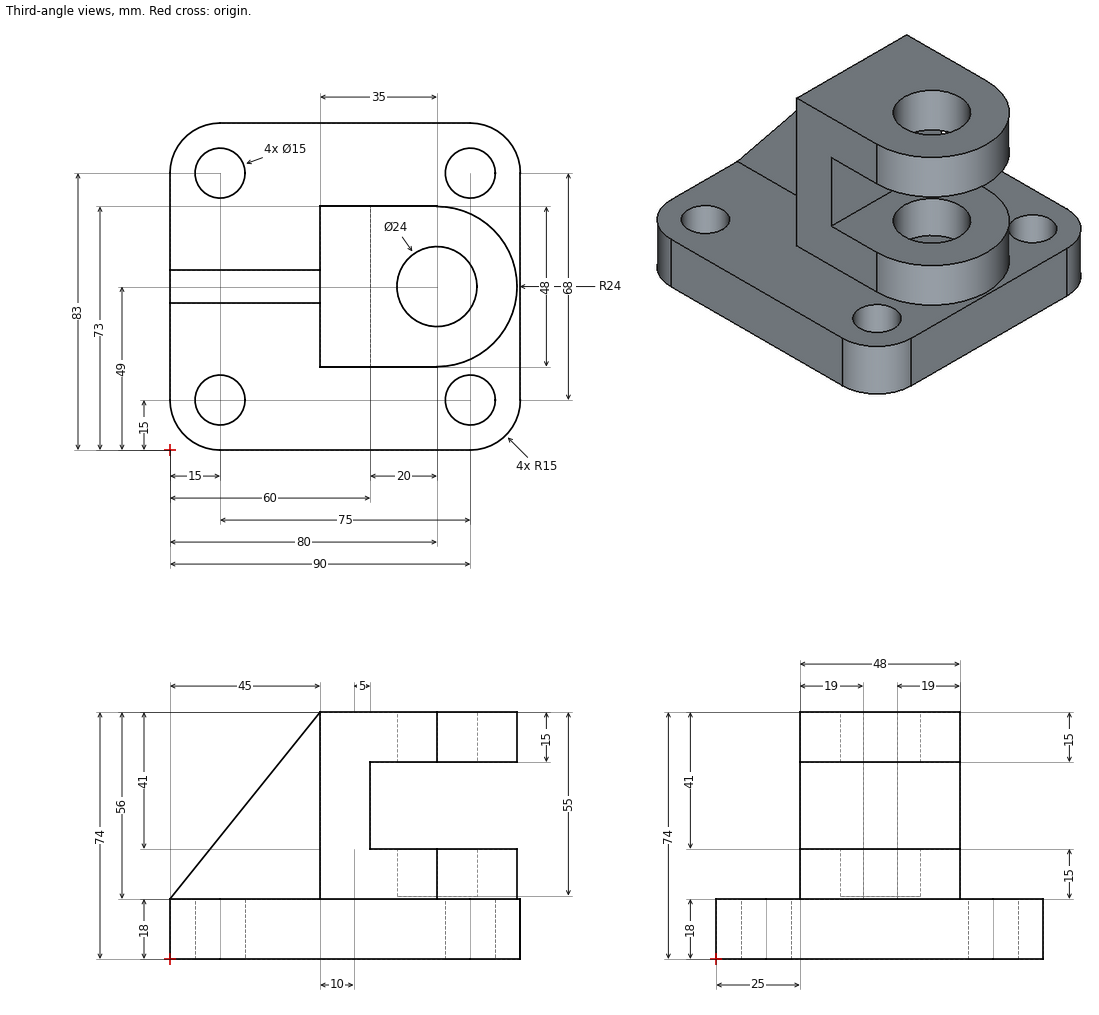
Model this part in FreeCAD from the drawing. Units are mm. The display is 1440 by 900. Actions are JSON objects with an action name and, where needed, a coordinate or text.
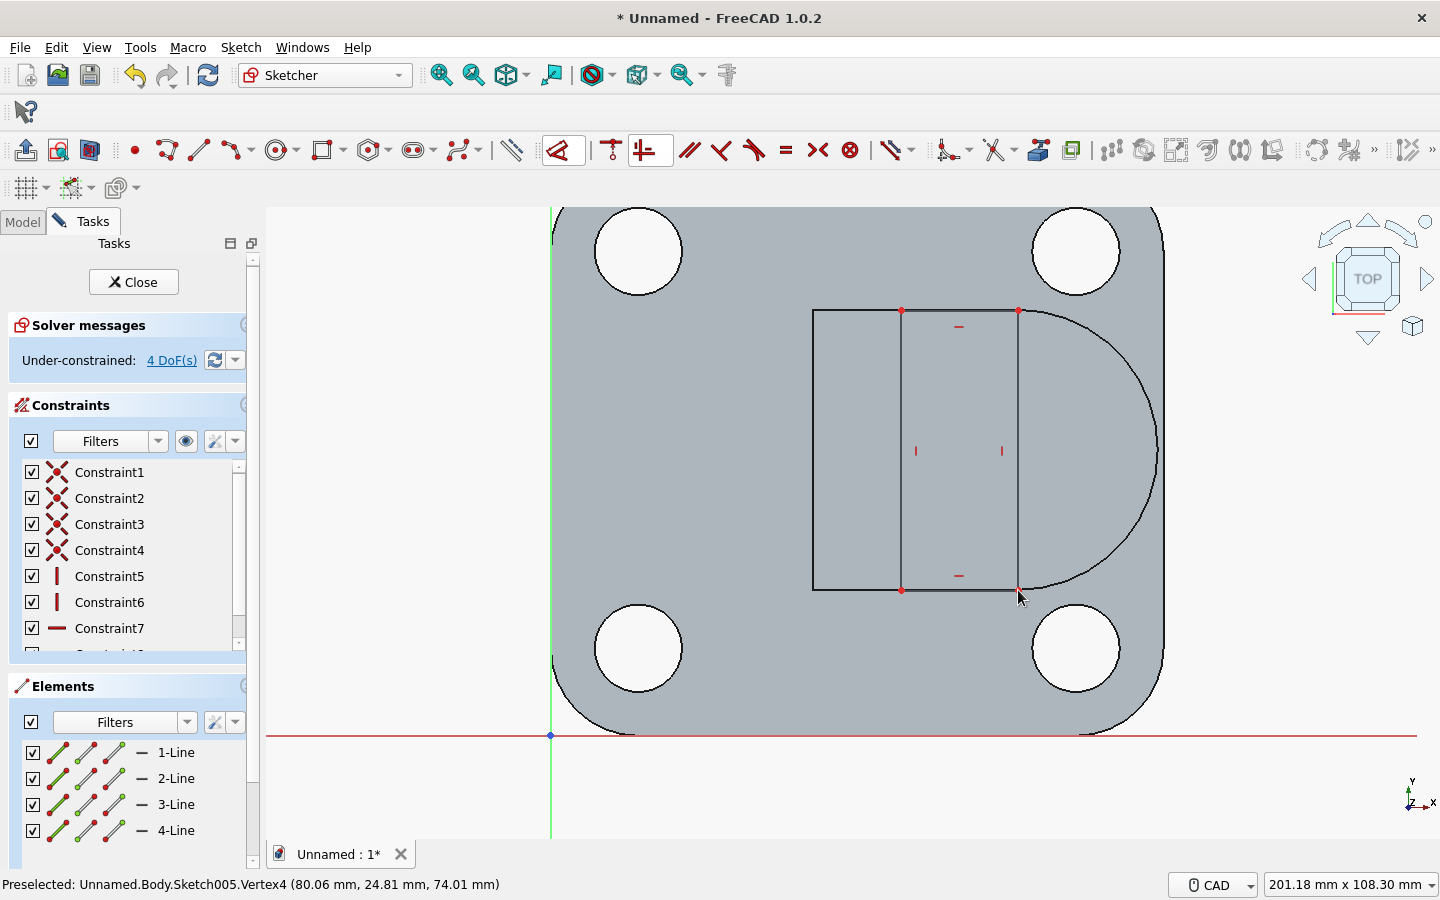
{"action": "left_click", "coordinate": [901, 395]}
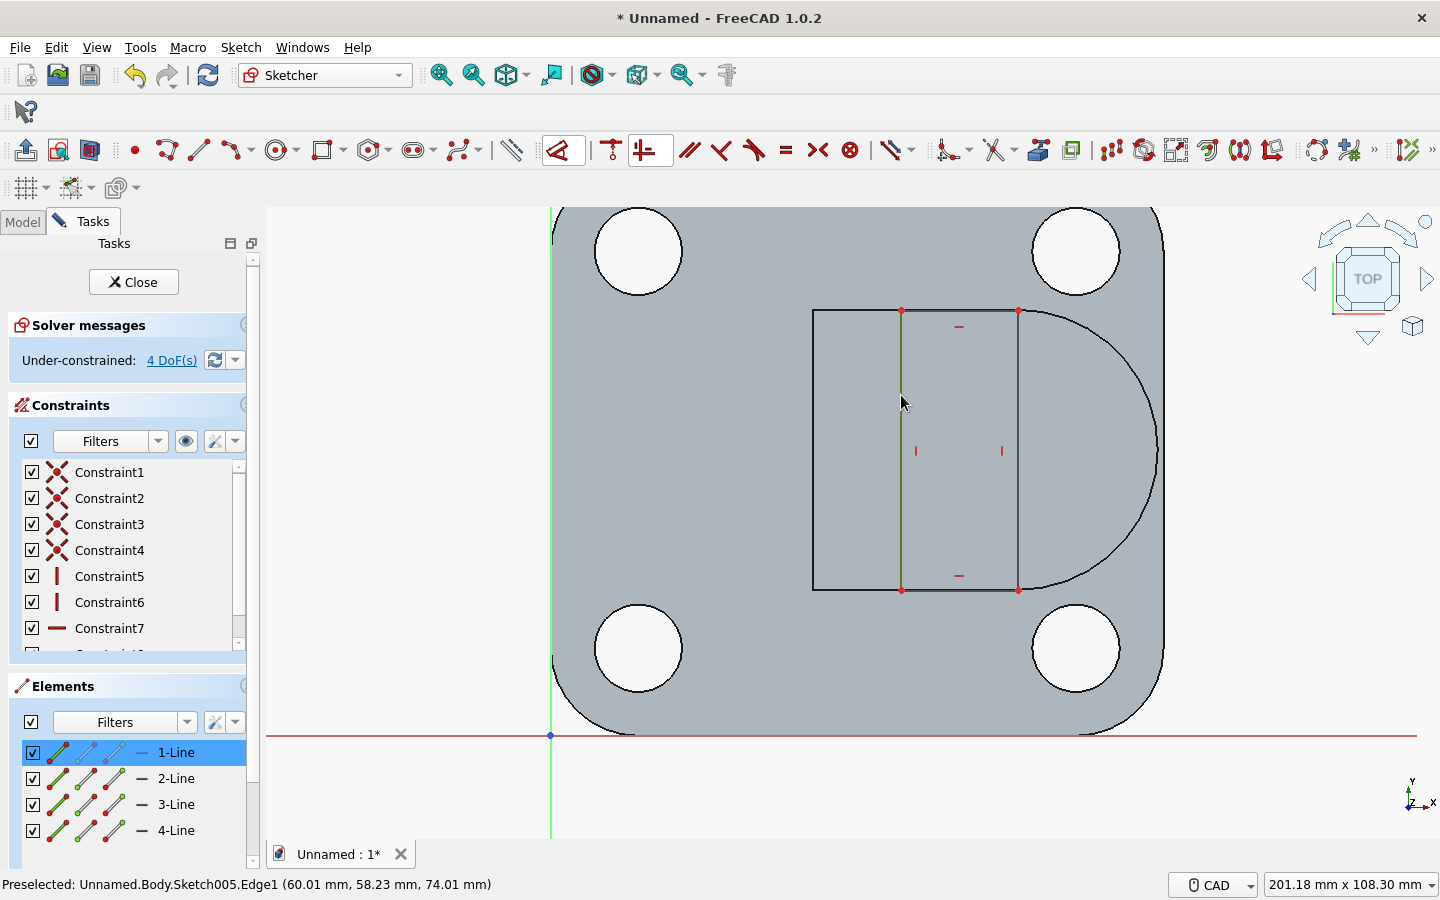
{"action": "left_click", "coordinate": [580, 150]}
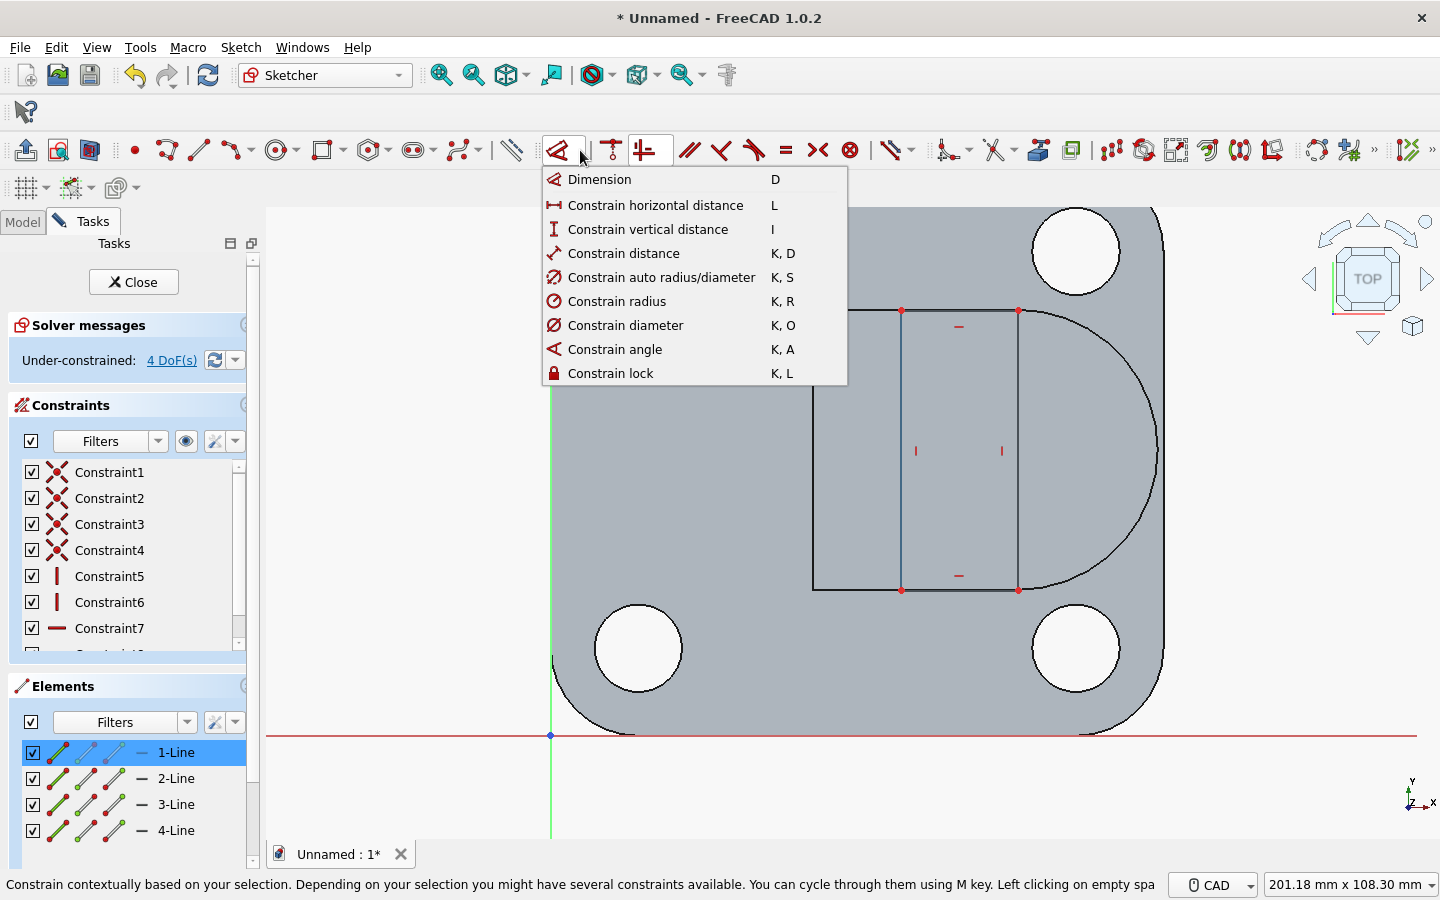
{"action": "left_click", "coordinate": [695, 229]}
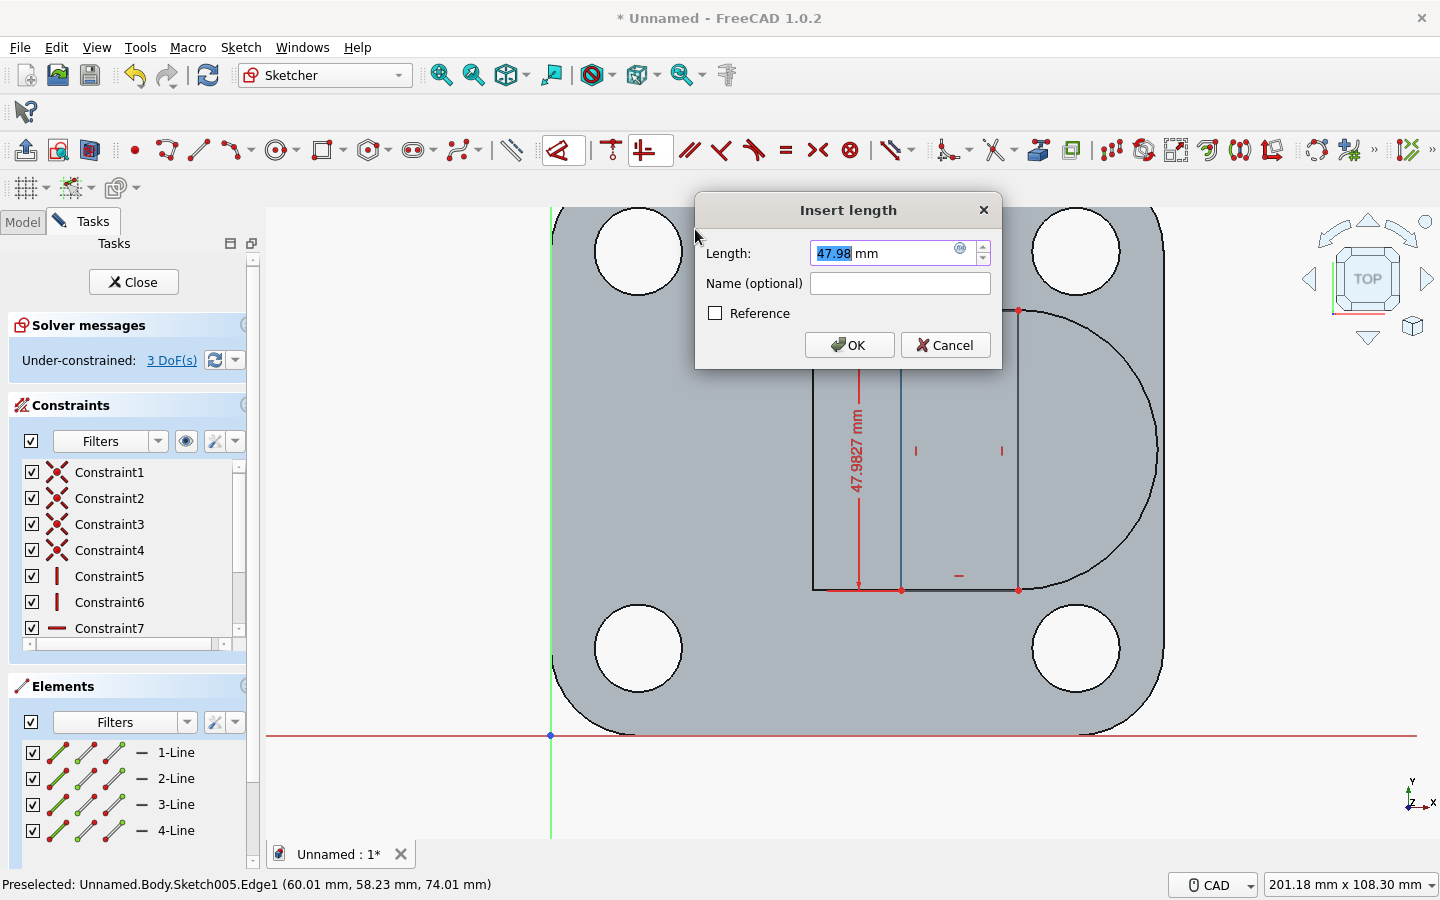
{"action": "type", "text": "48"}
{"action": "key", "text": "Return"}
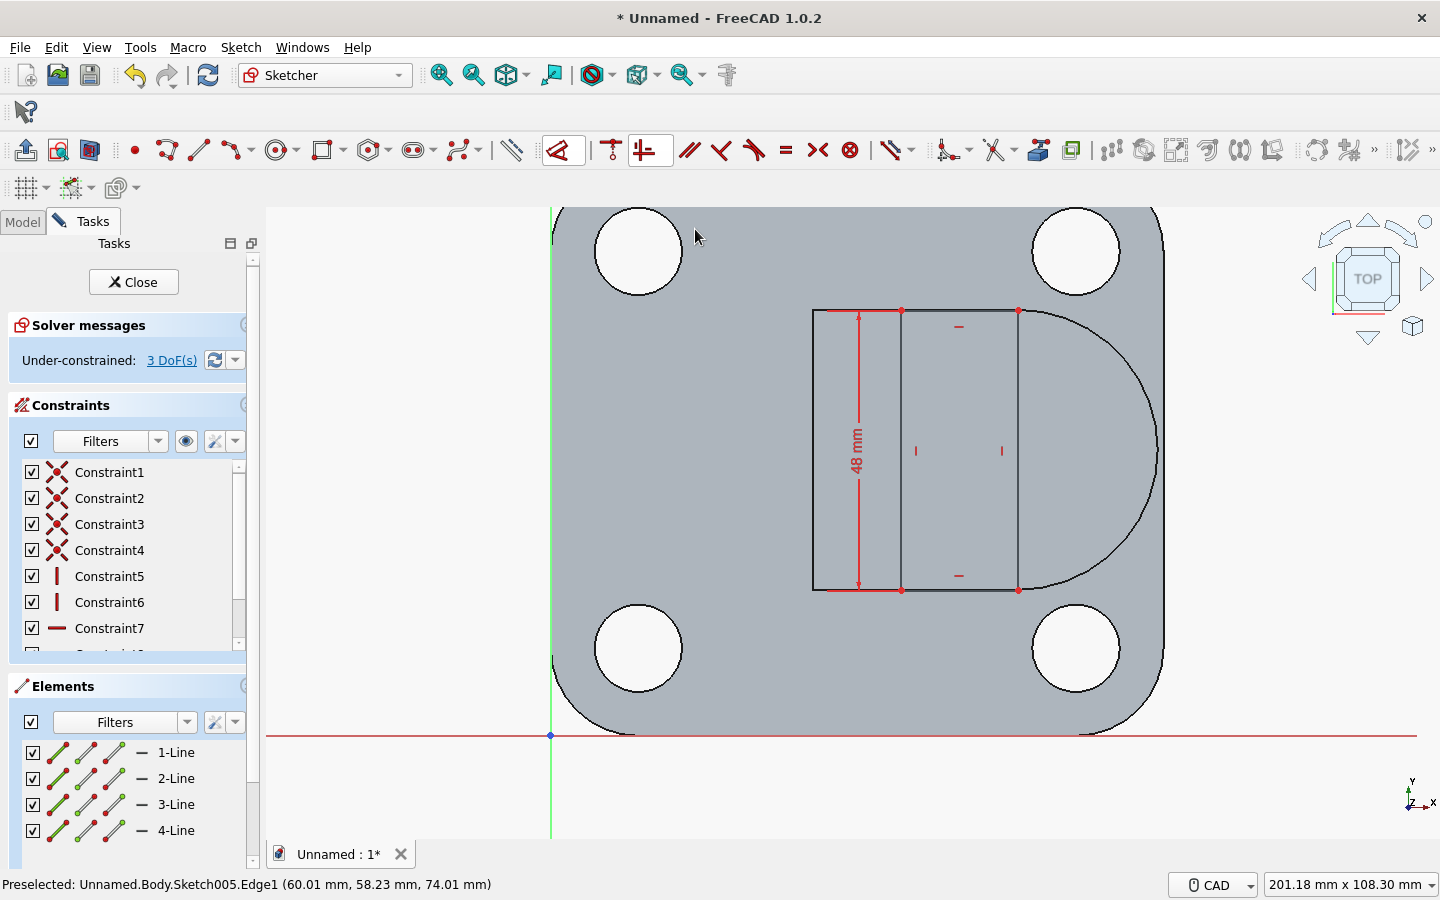
{"action": "left_click", "coordinate": [936, 591]}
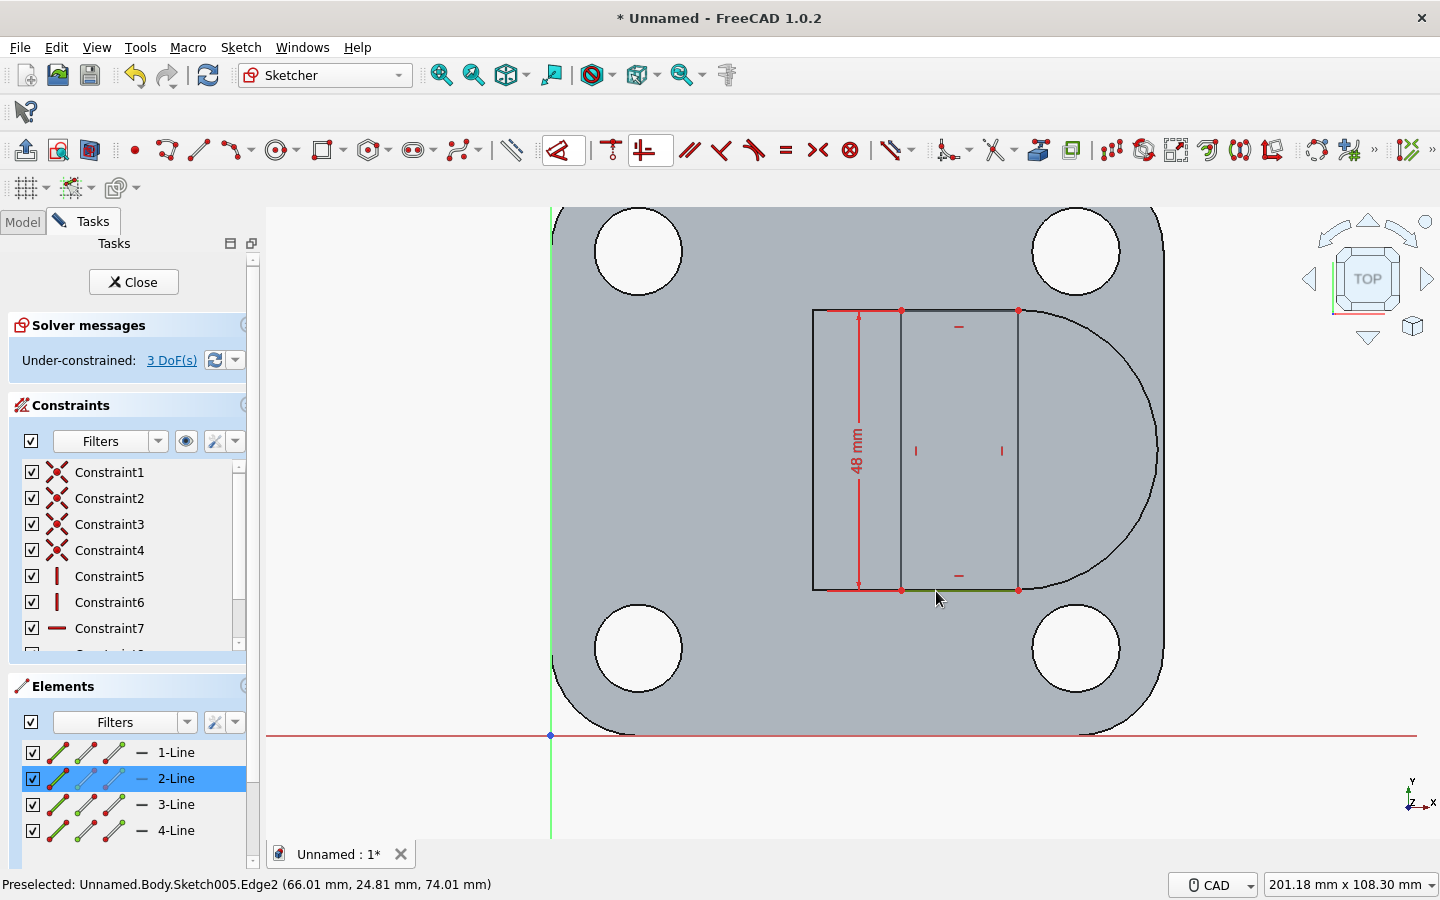
{"action": "left_click", "coordinate": [580, 150]}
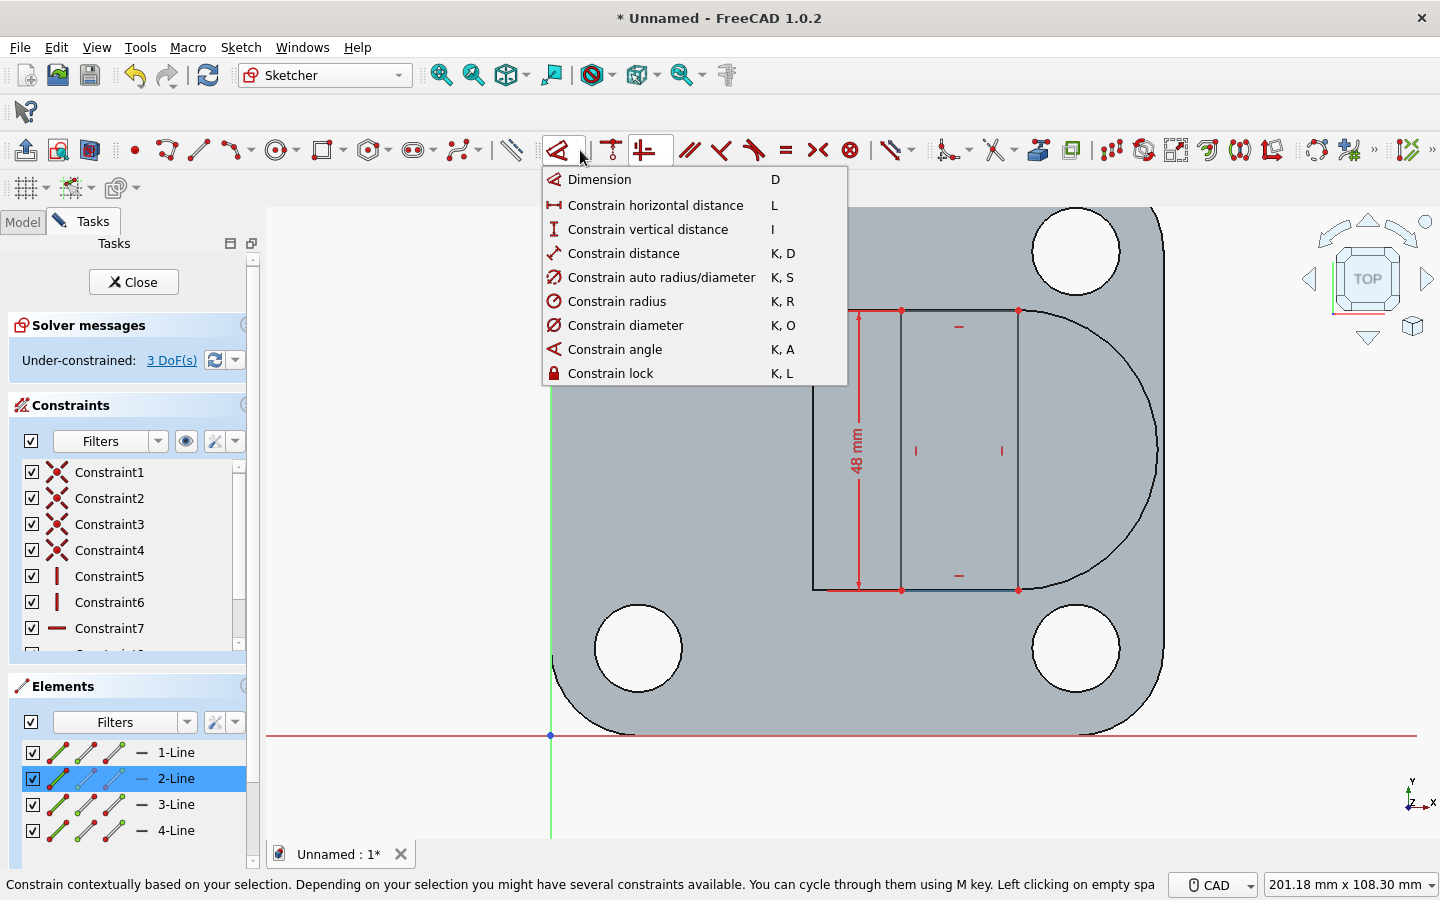
{"action": "left_click", "coordinate": [695, 205]}